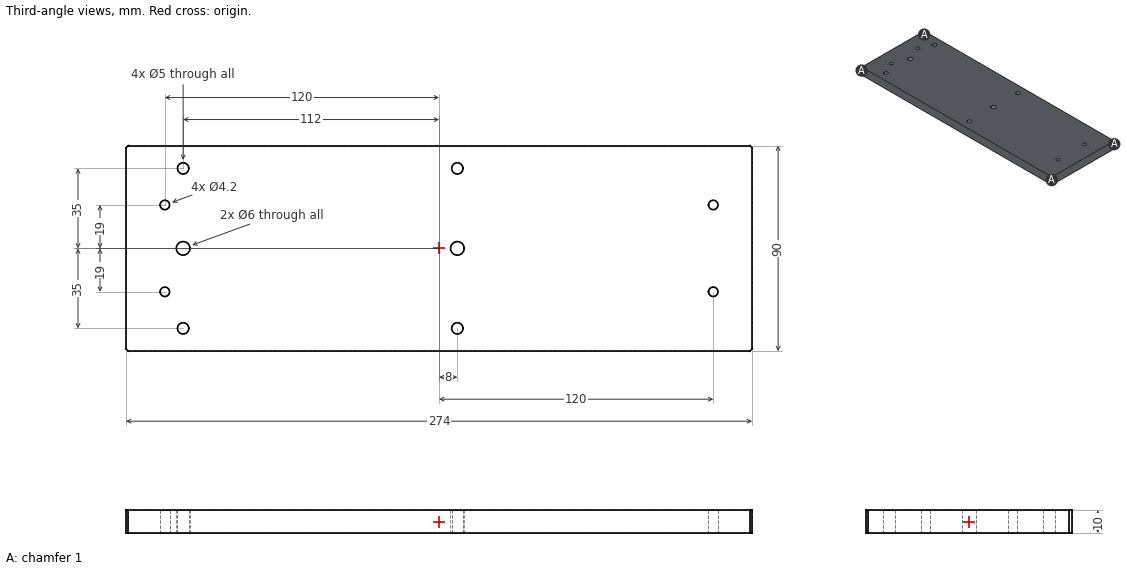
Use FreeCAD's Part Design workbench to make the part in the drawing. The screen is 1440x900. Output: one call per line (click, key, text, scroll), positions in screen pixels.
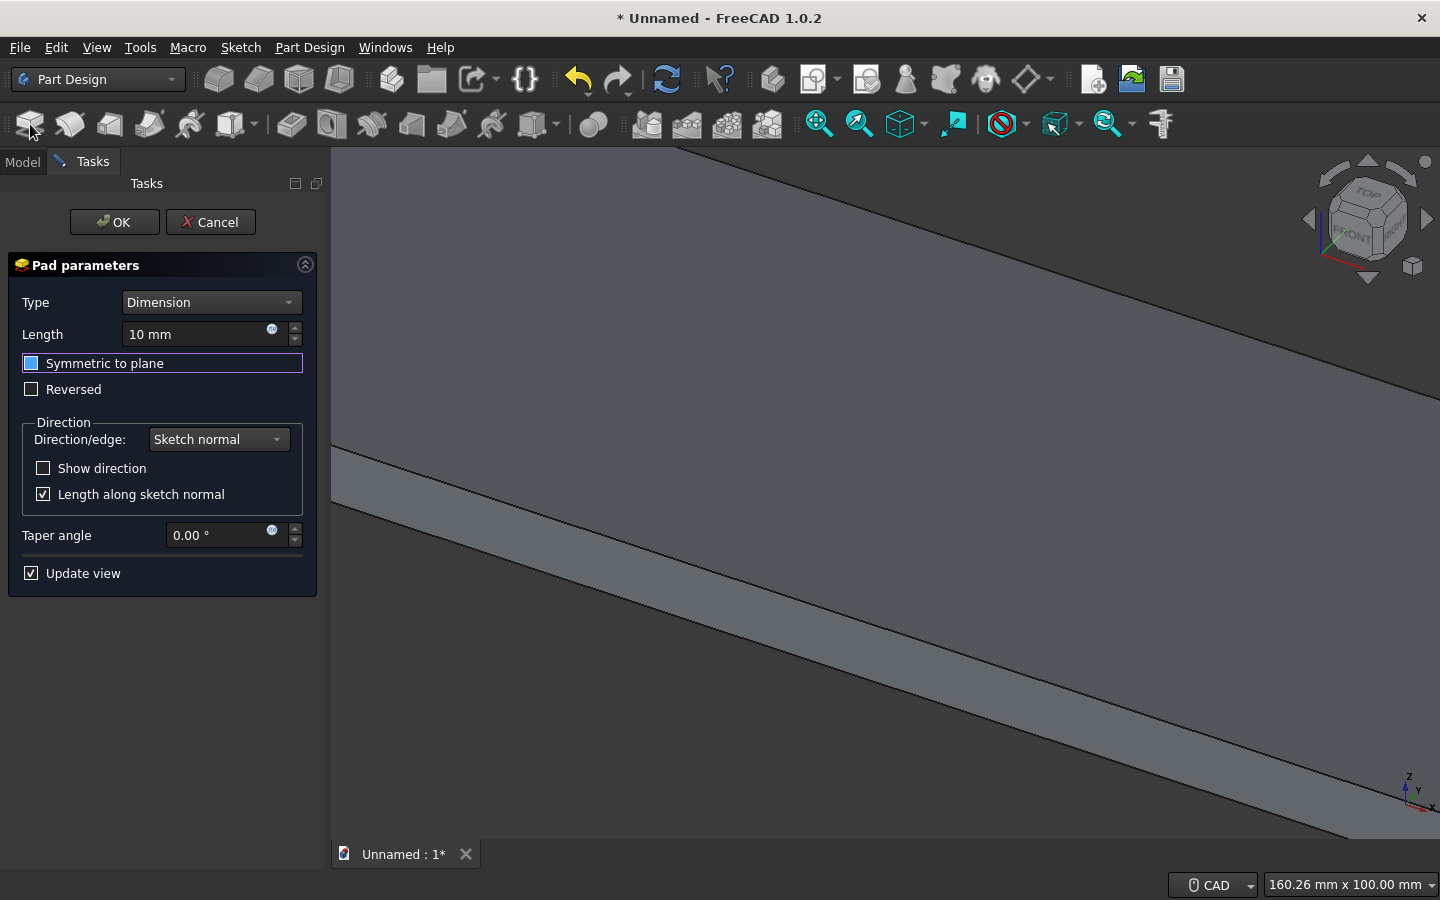
click(30, 363)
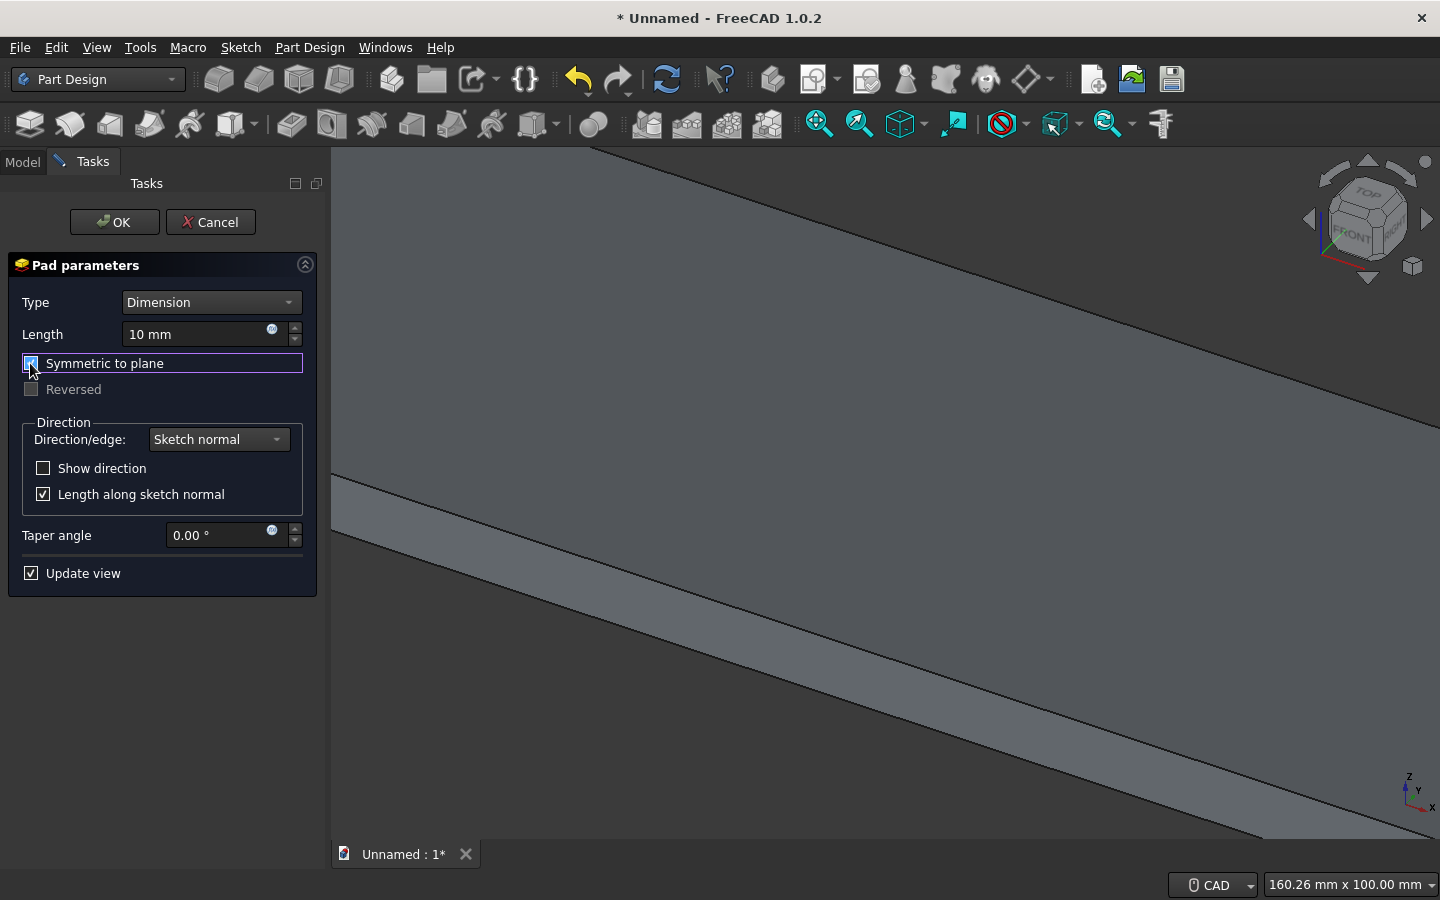
click(115, 222)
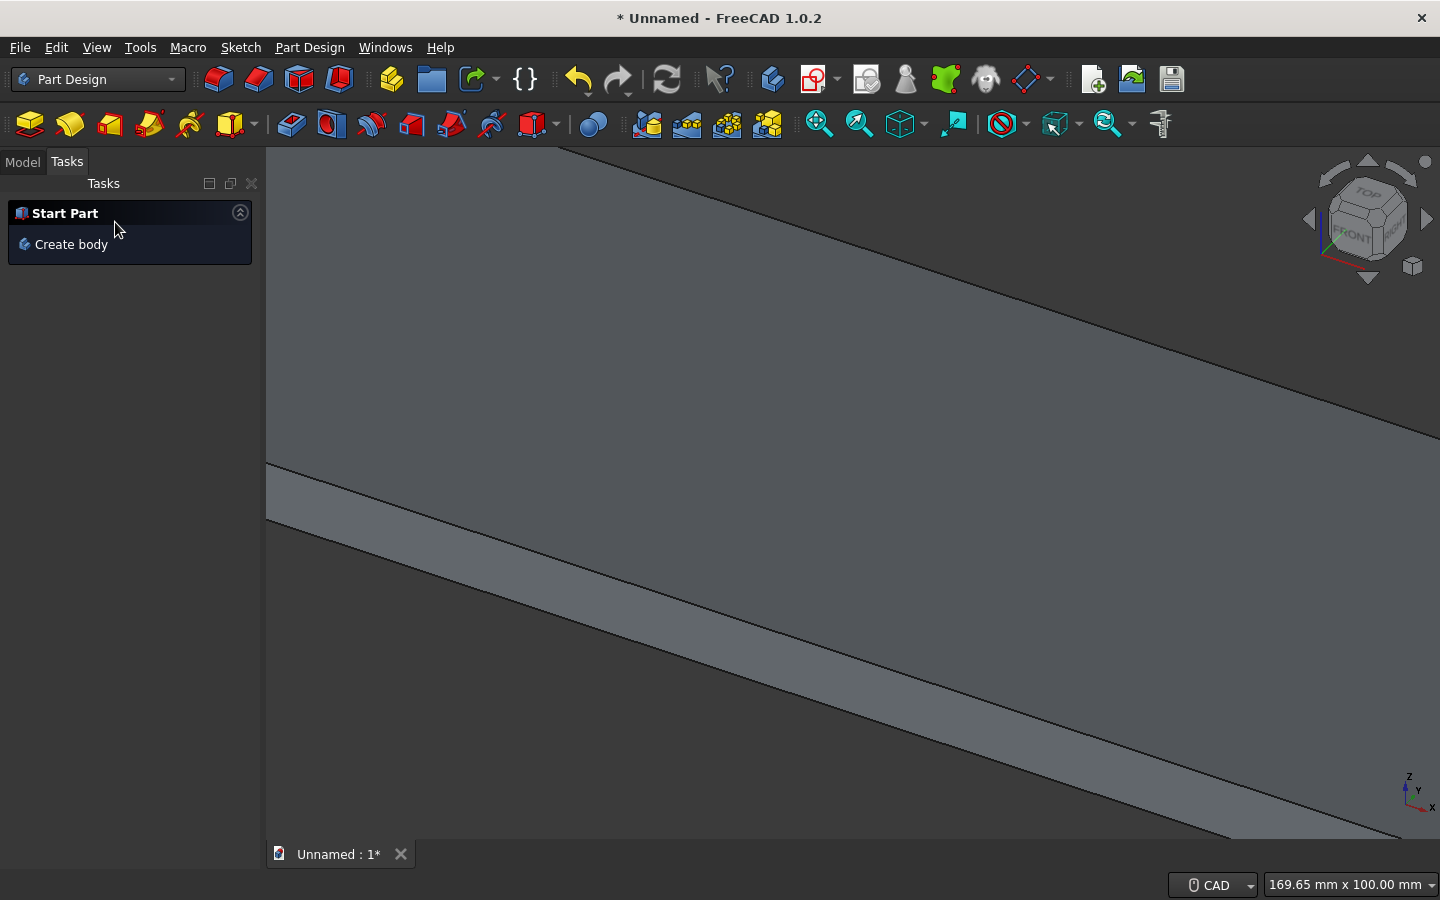
click(820, 124)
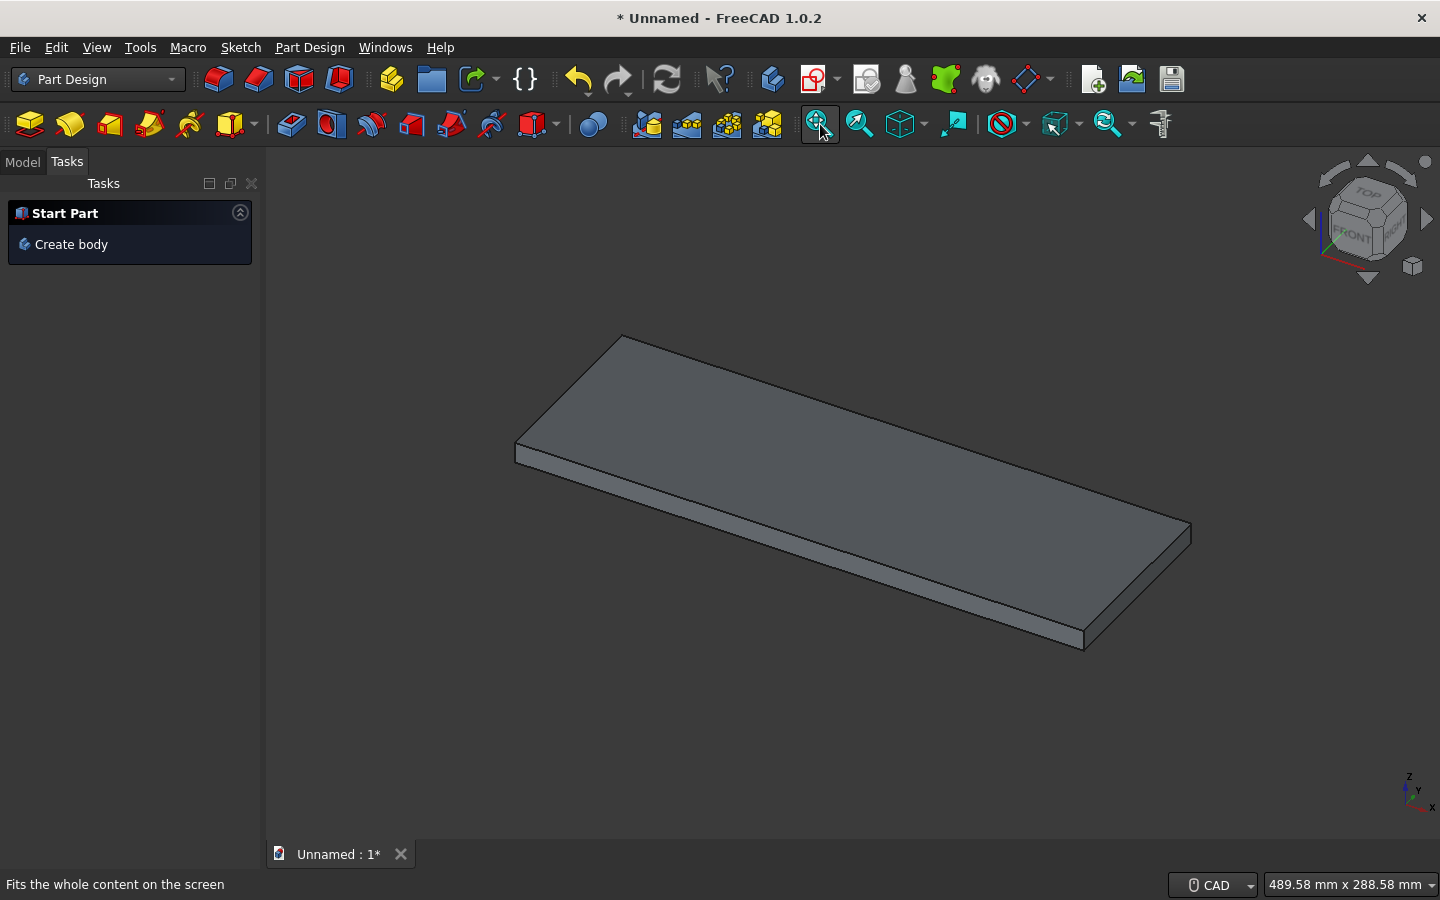
click(1016, 536)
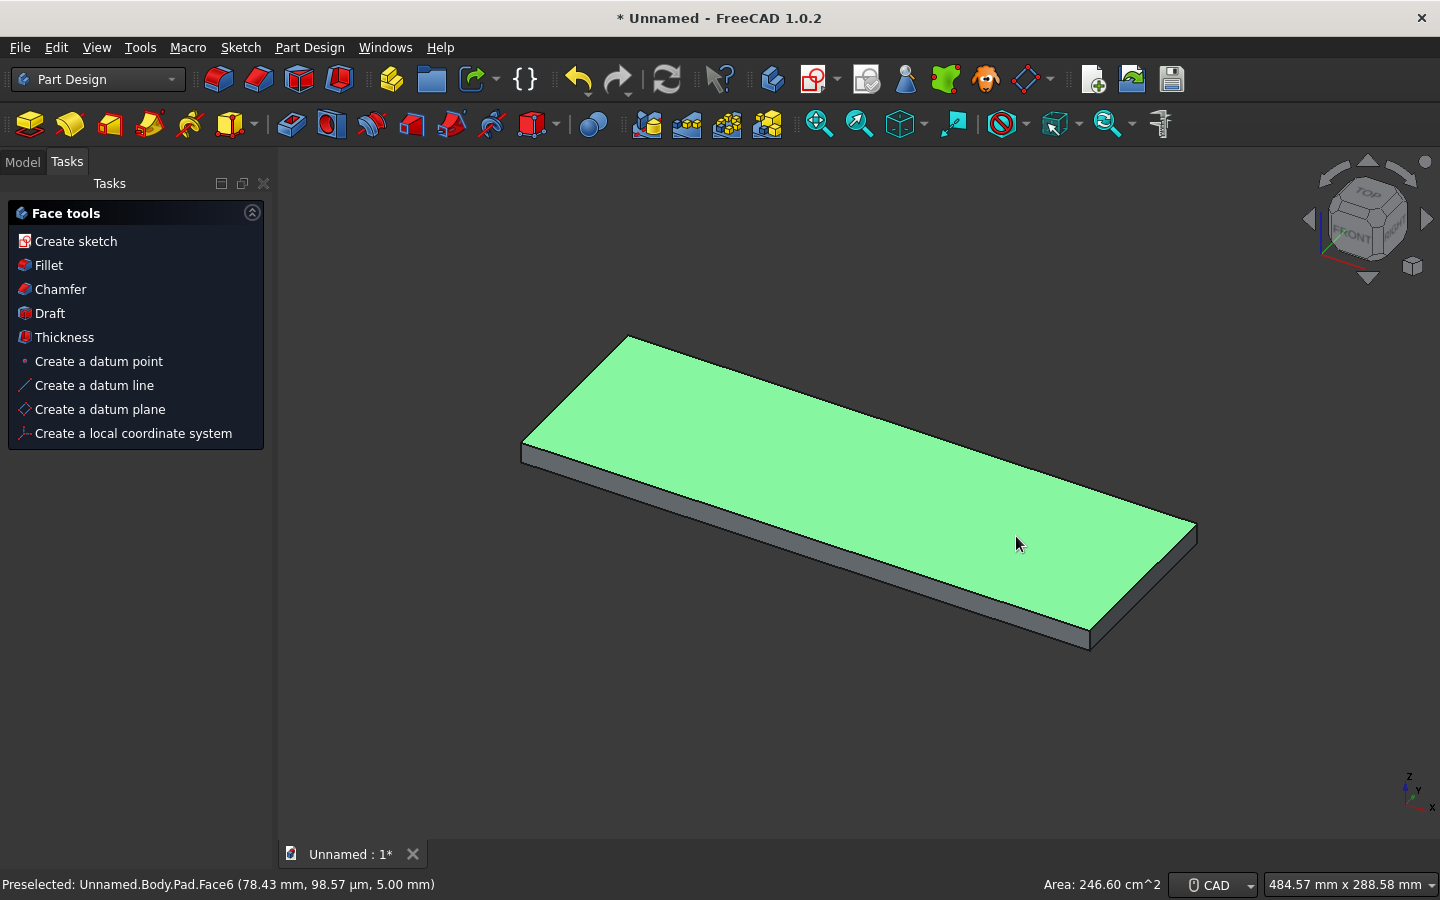
click(814, 80)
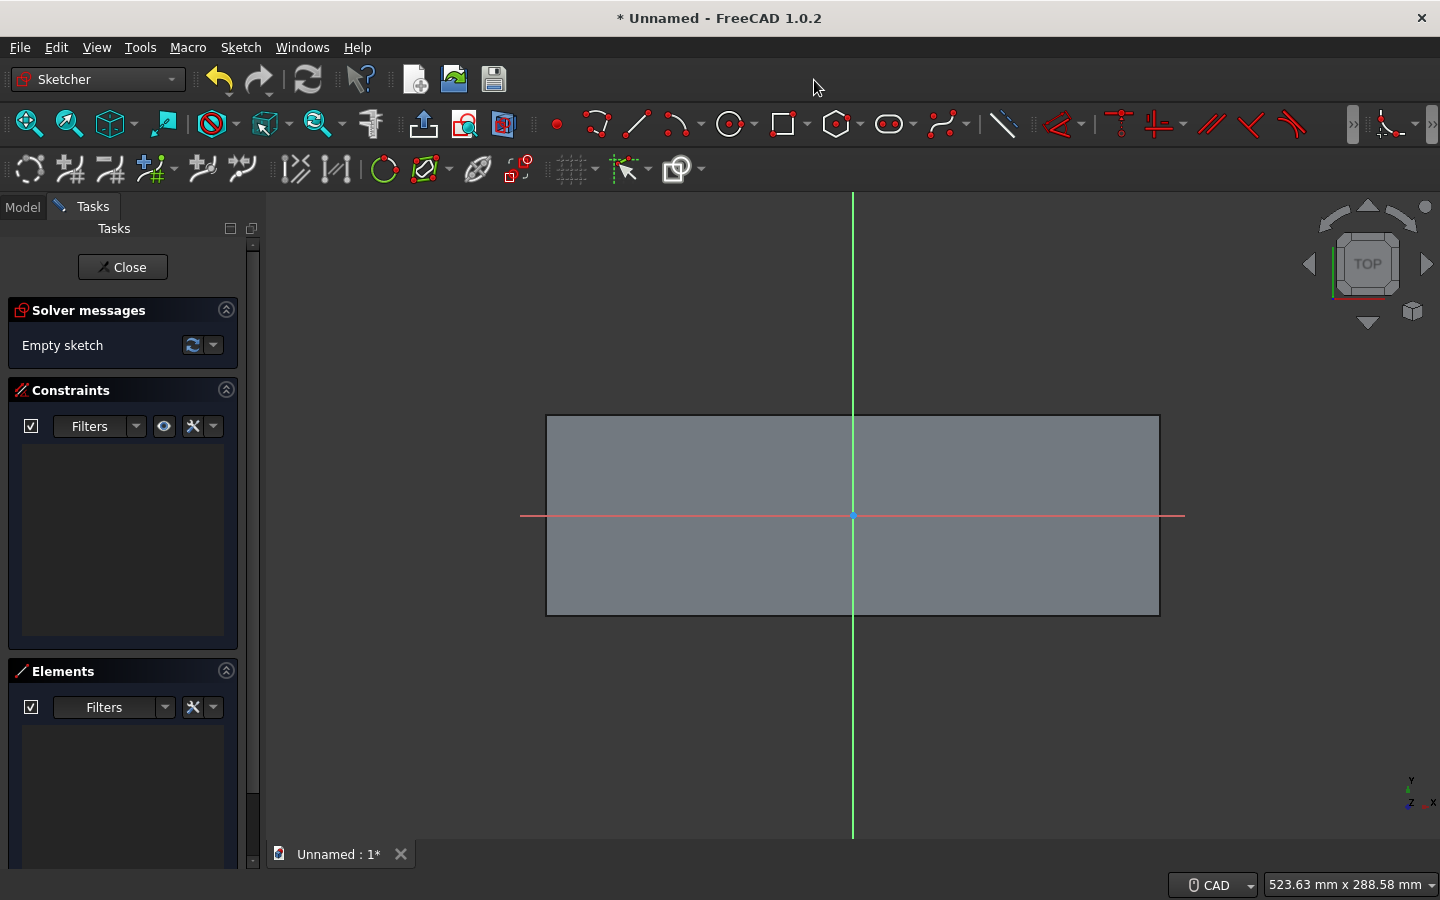
key(g)
key(c)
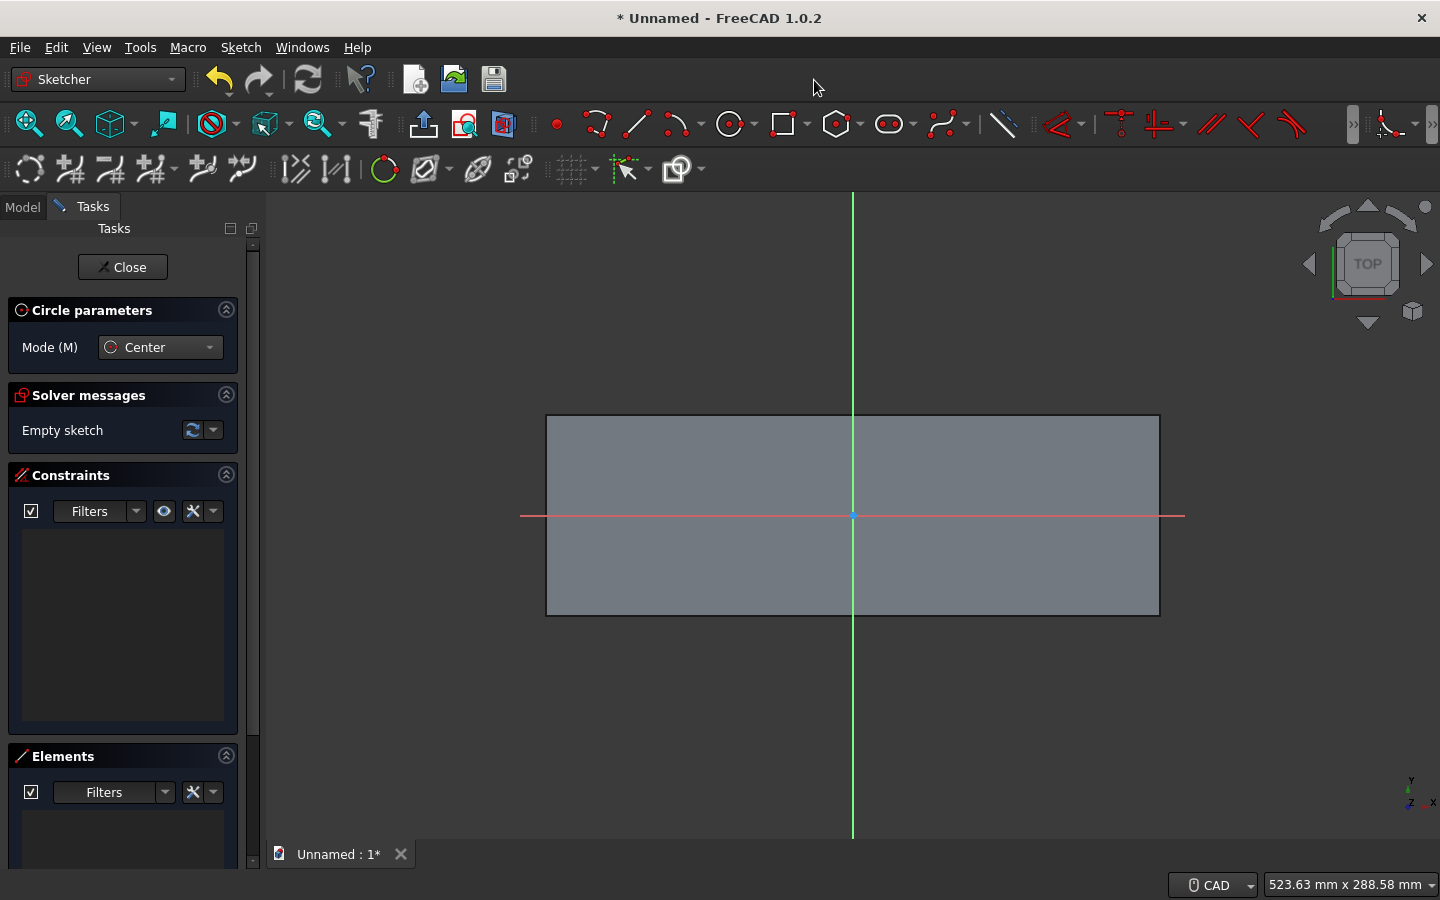
scroll(584, 473, up, 8)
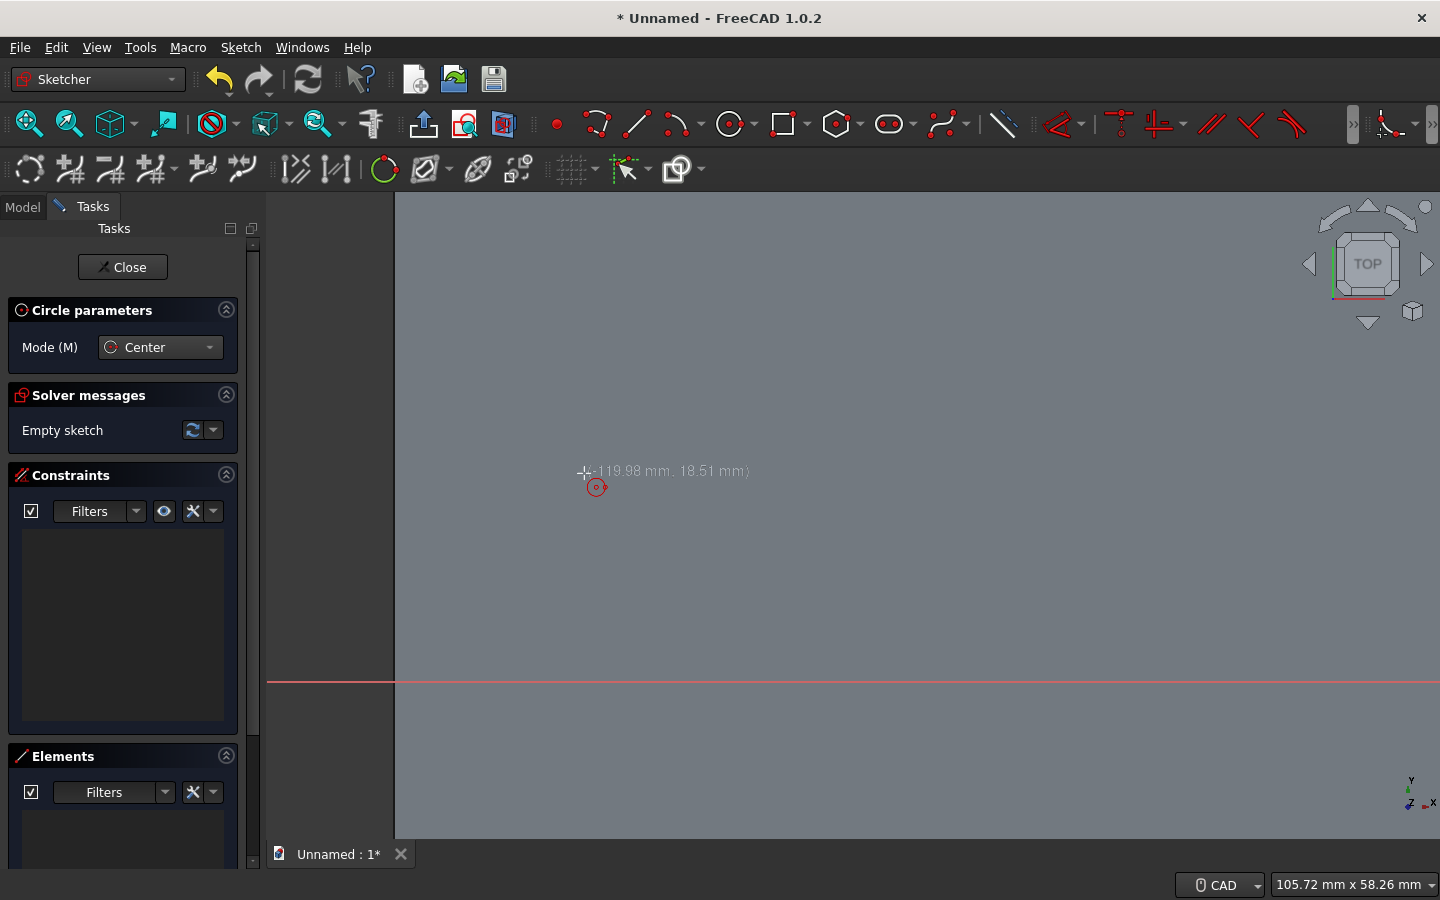
scroll(414, 461, down, 7)